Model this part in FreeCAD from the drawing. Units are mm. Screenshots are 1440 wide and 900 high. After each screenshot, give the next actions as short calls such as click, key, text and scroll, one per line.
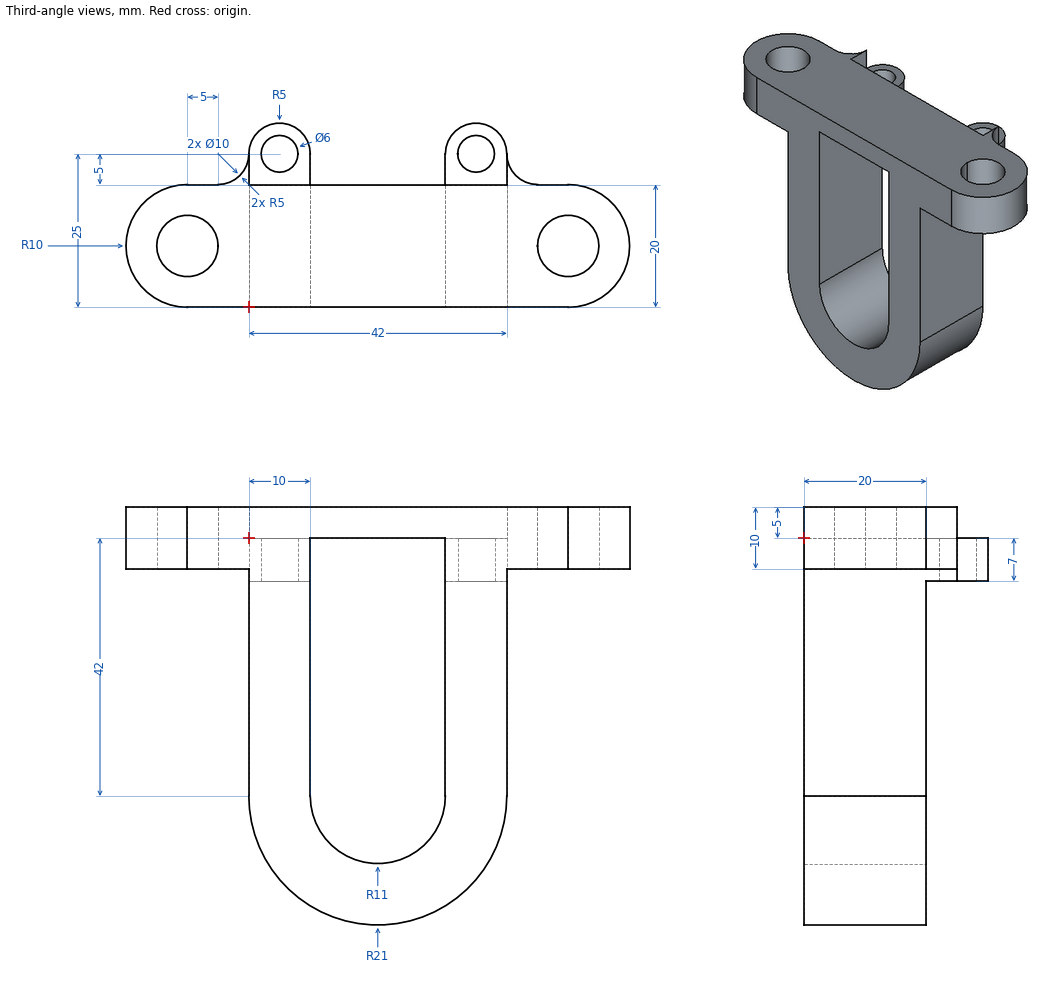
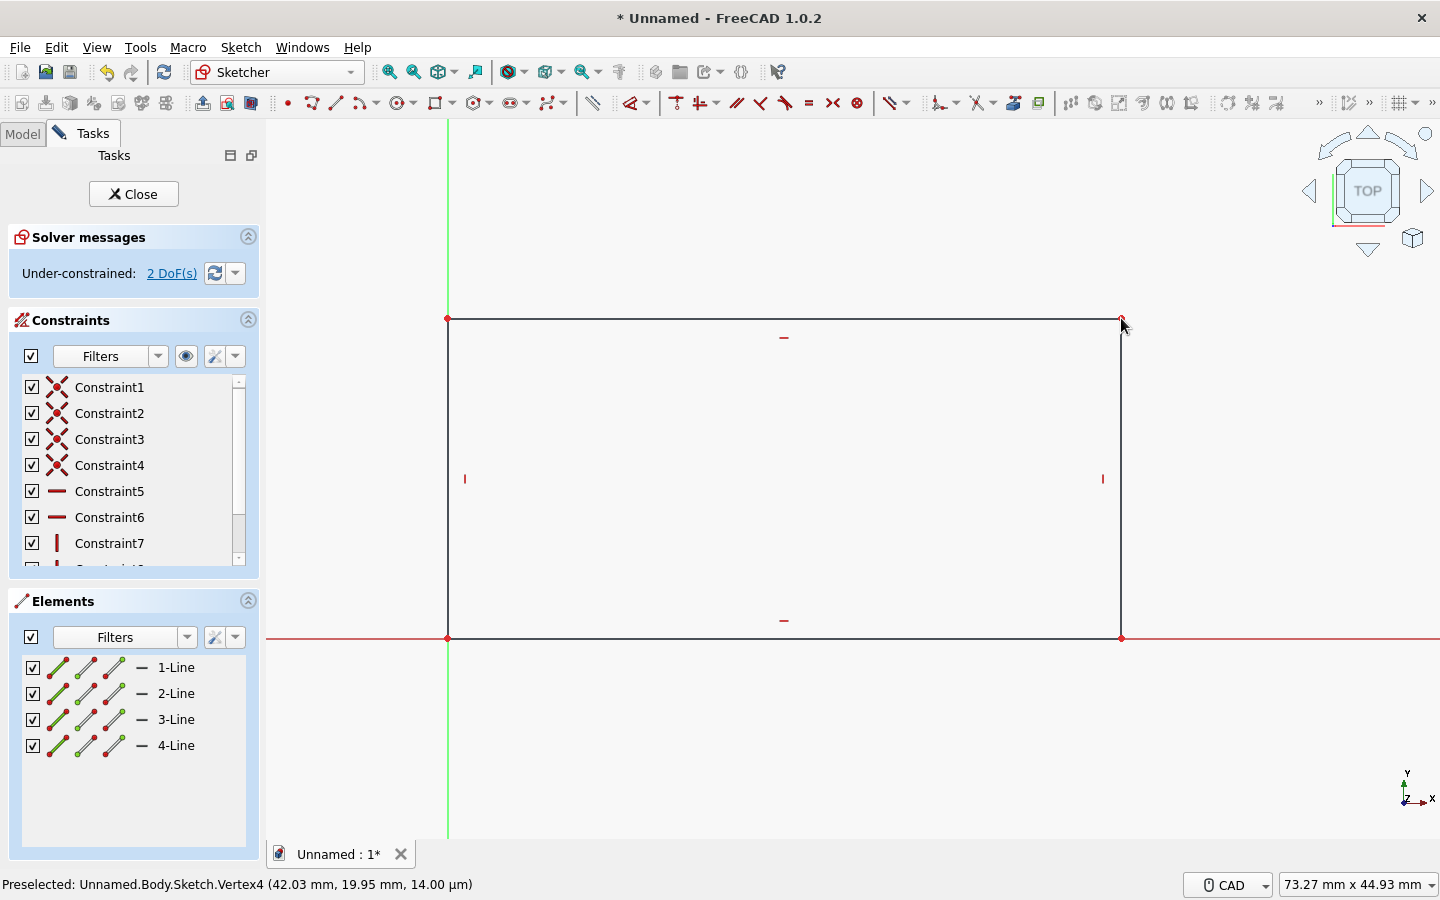
click(630, 104)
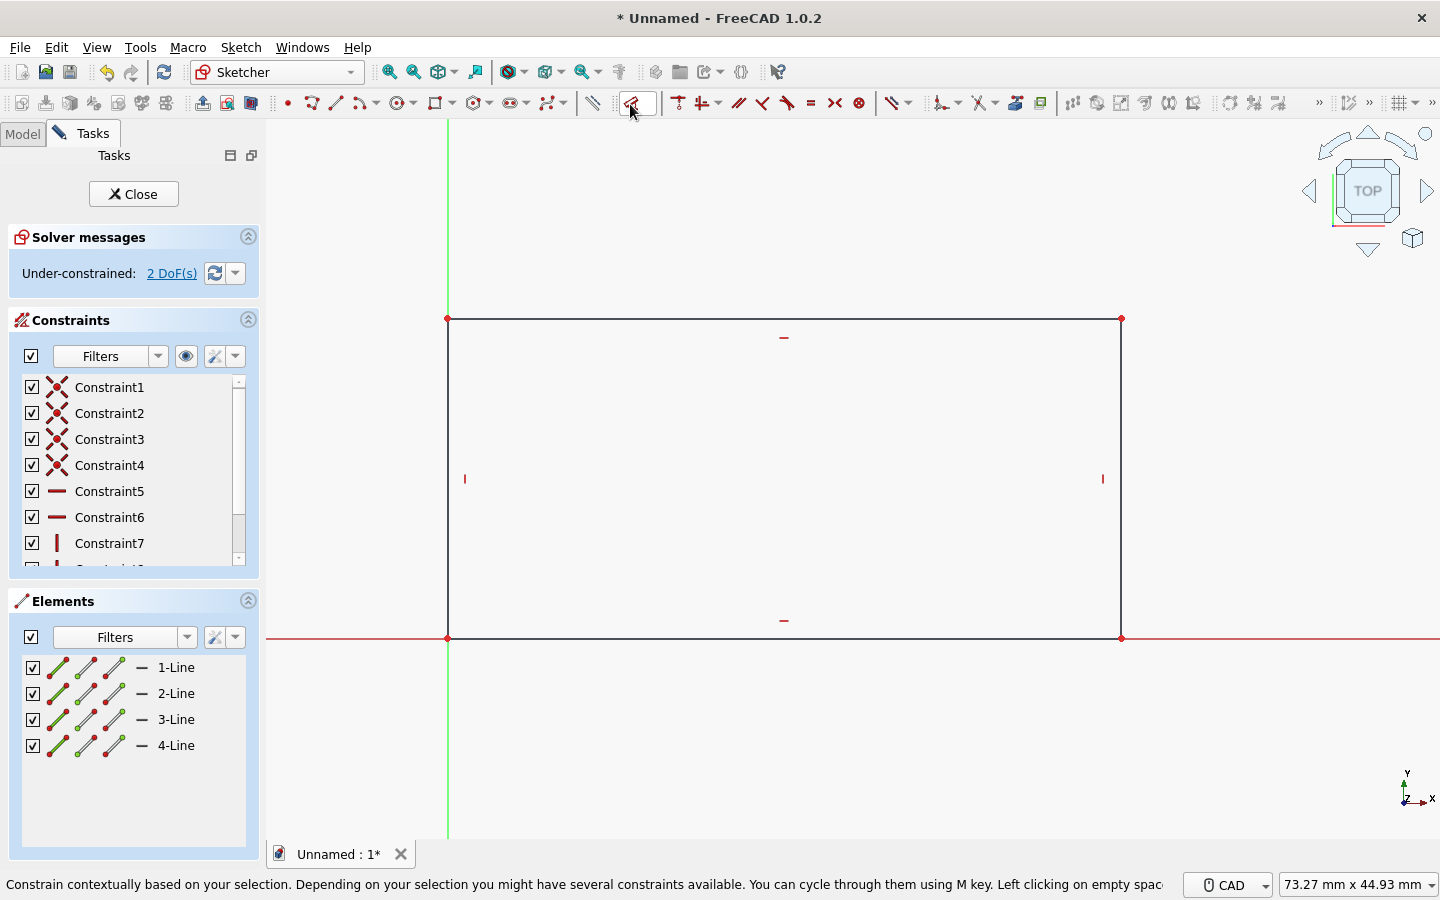
click(650, 639)
click(784, 673)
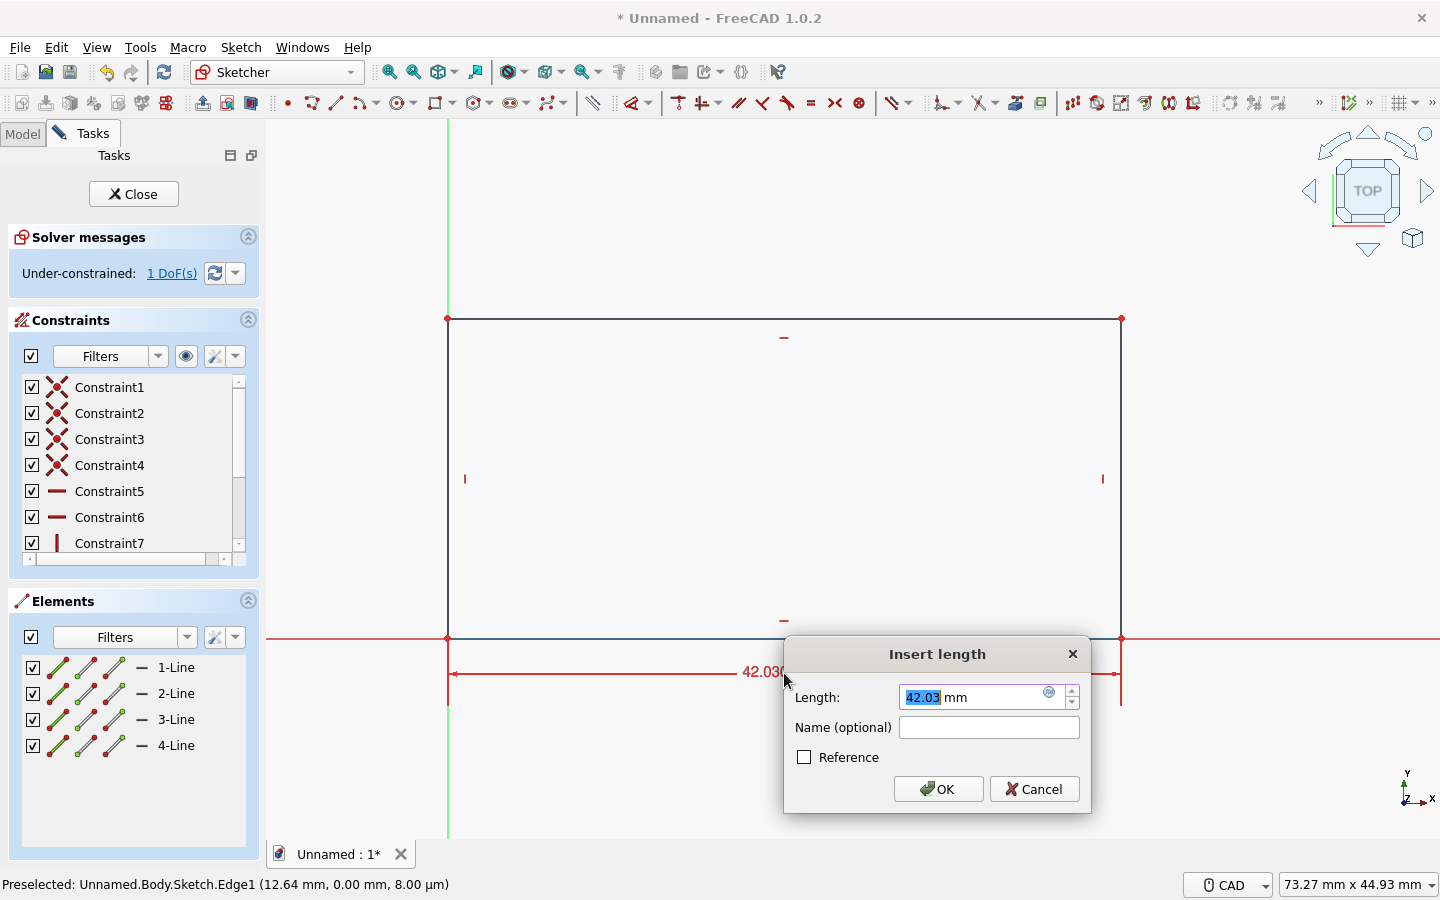
text(42)
key(Return)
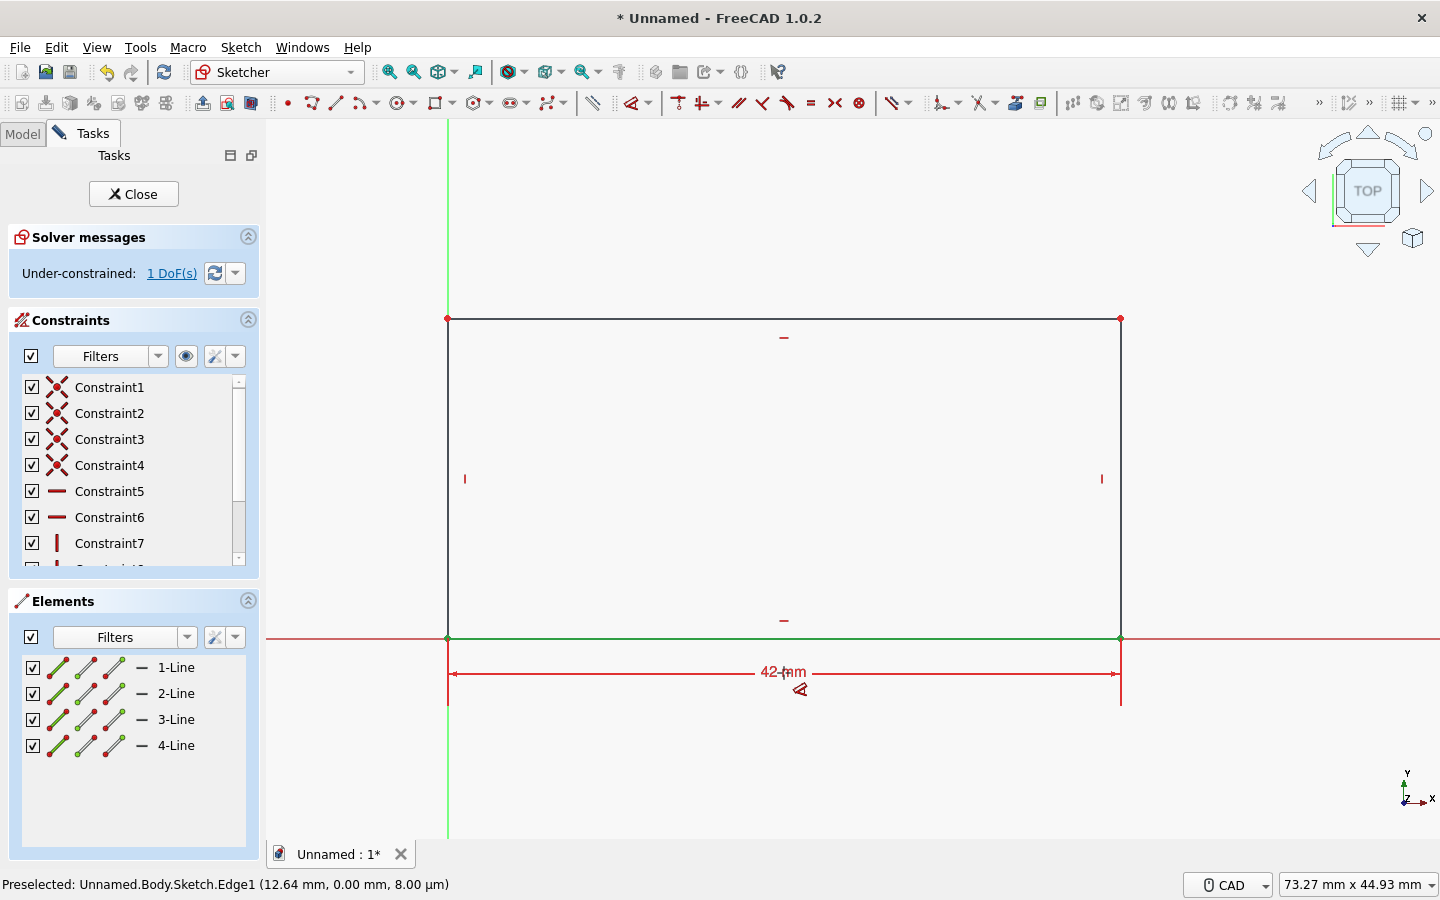
click(1121, 543)
click(1155, 479)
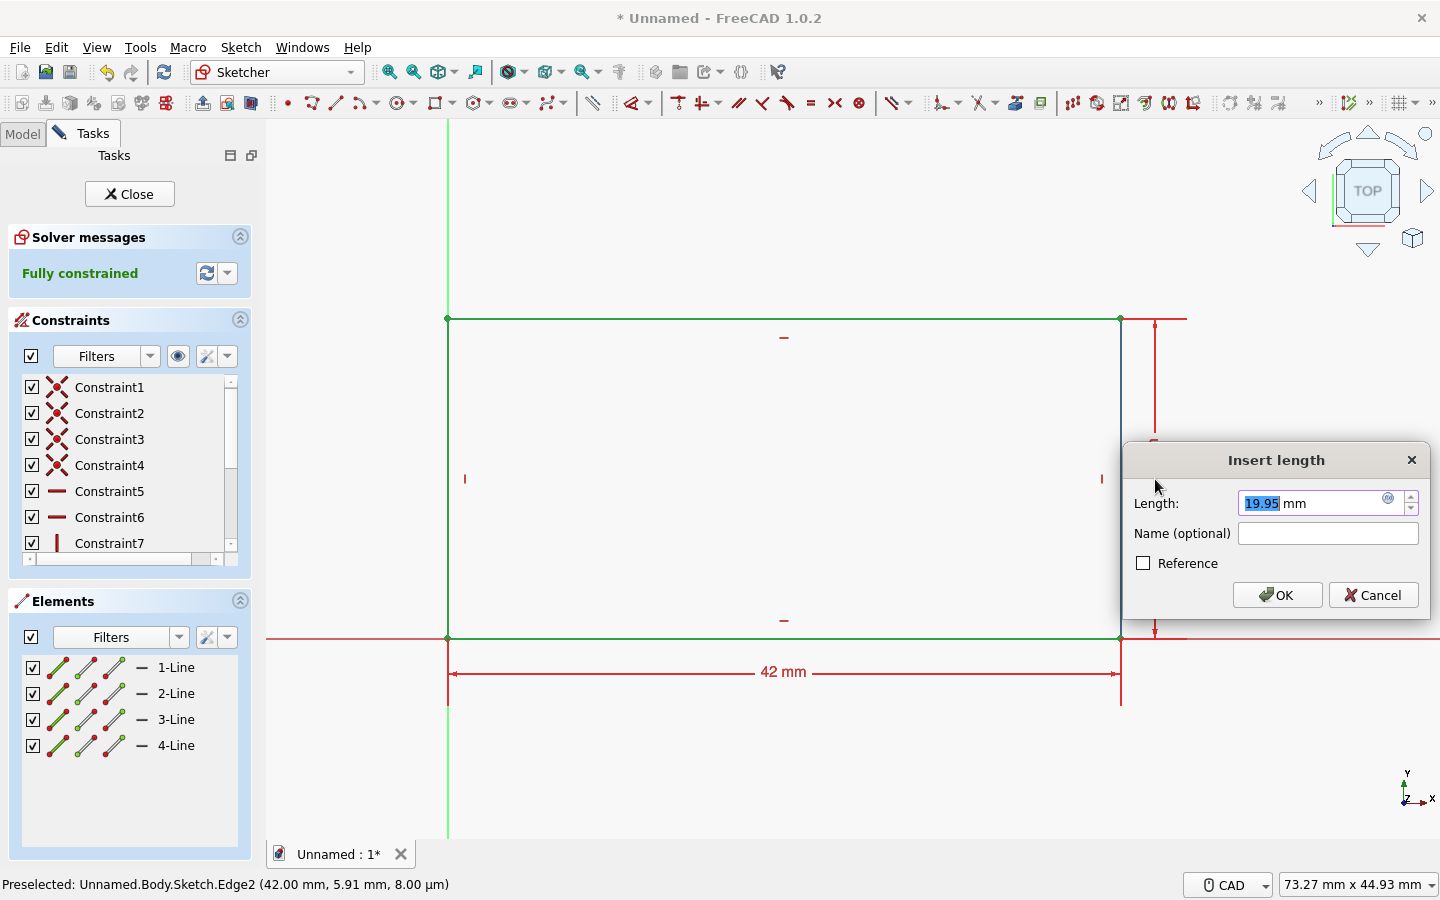
text(20)
key(Return)
key(Escape)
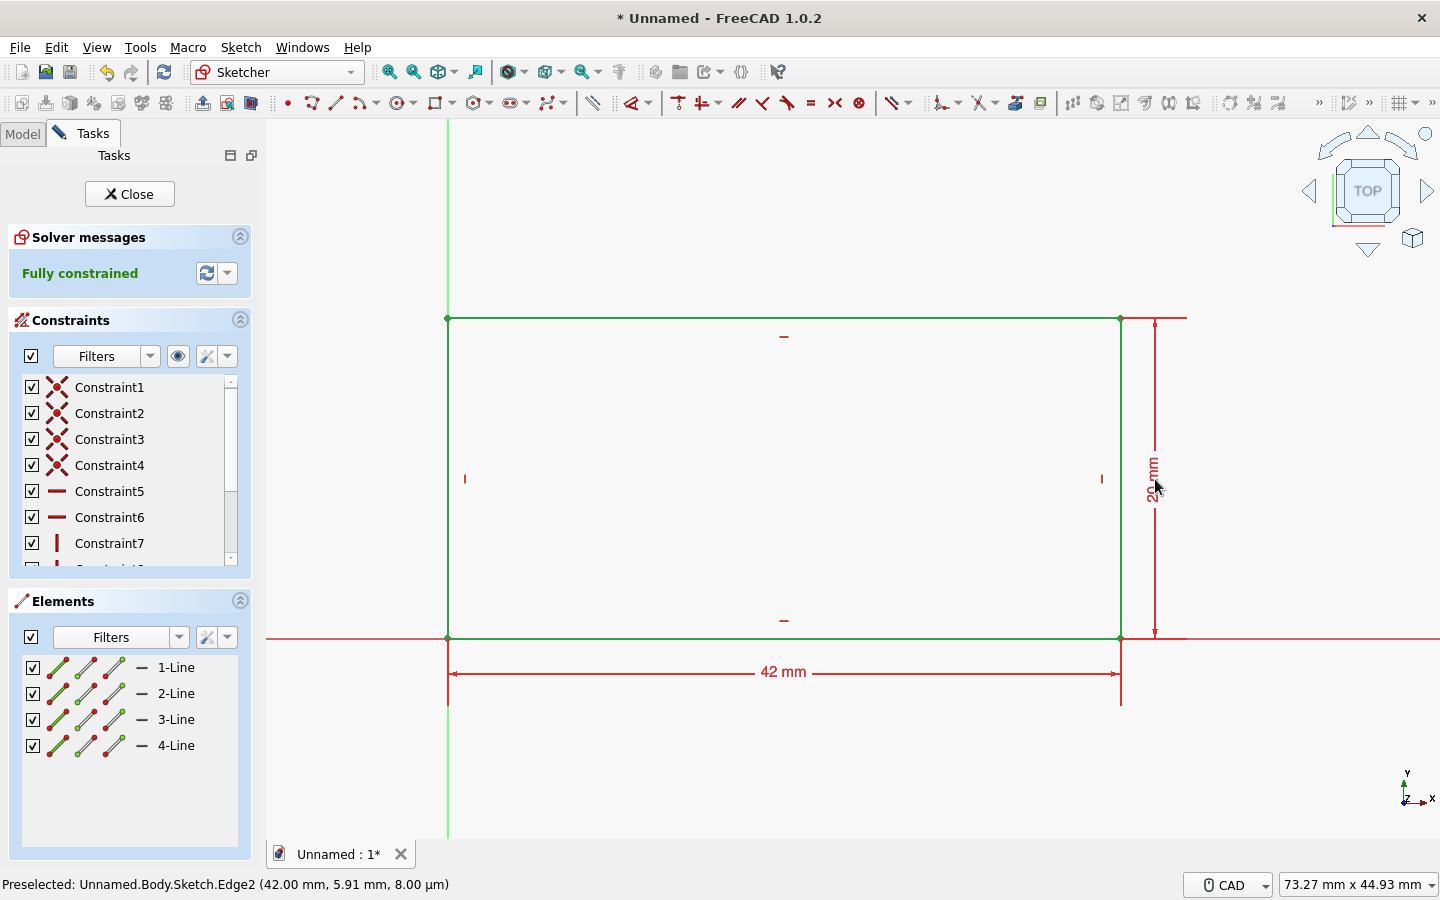
click(130, 194)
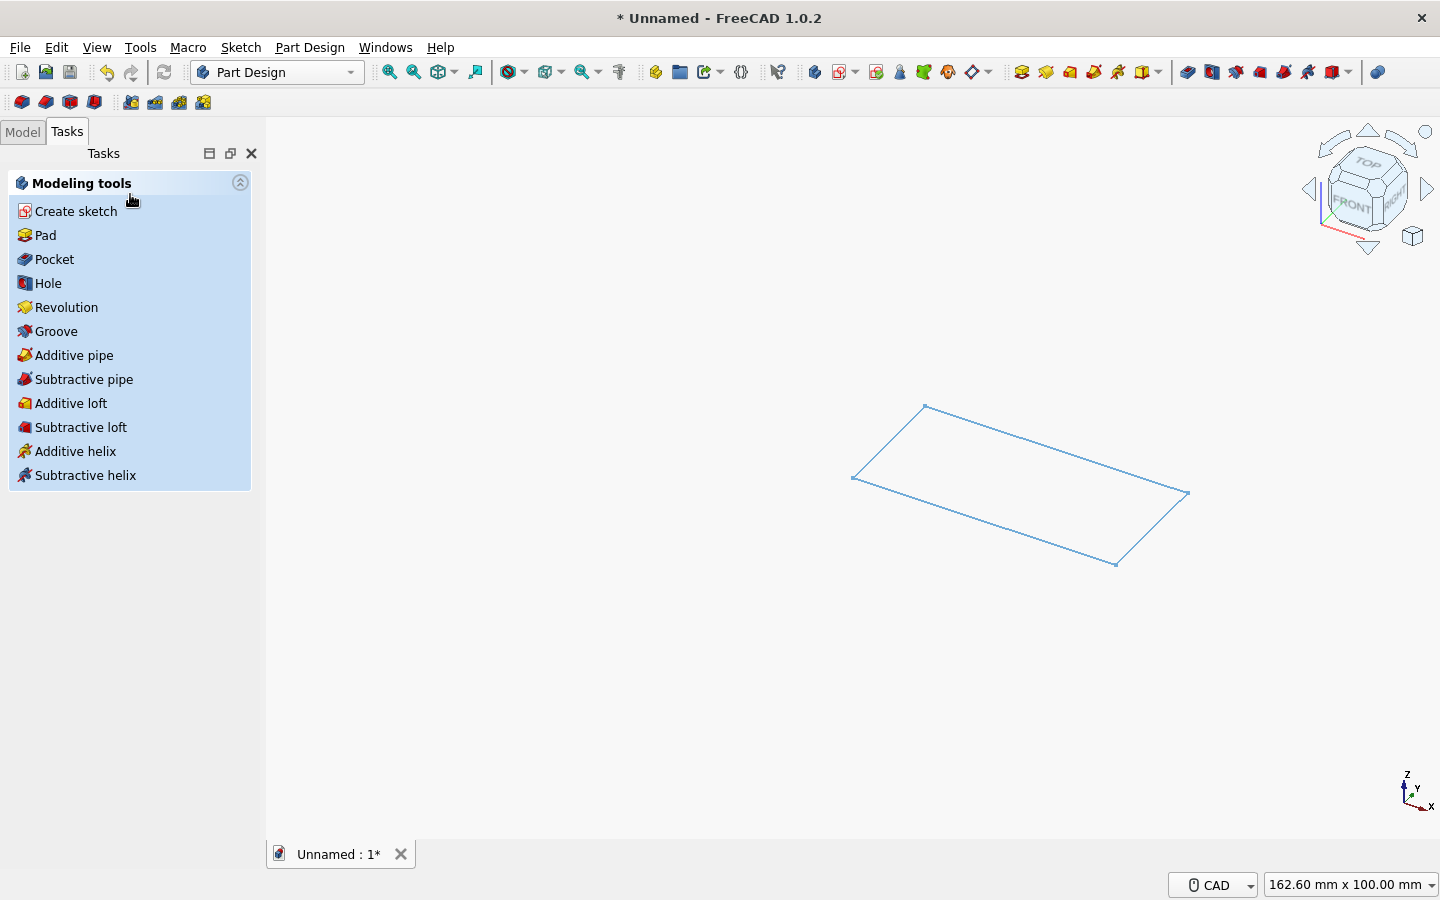
click(1022, 72)